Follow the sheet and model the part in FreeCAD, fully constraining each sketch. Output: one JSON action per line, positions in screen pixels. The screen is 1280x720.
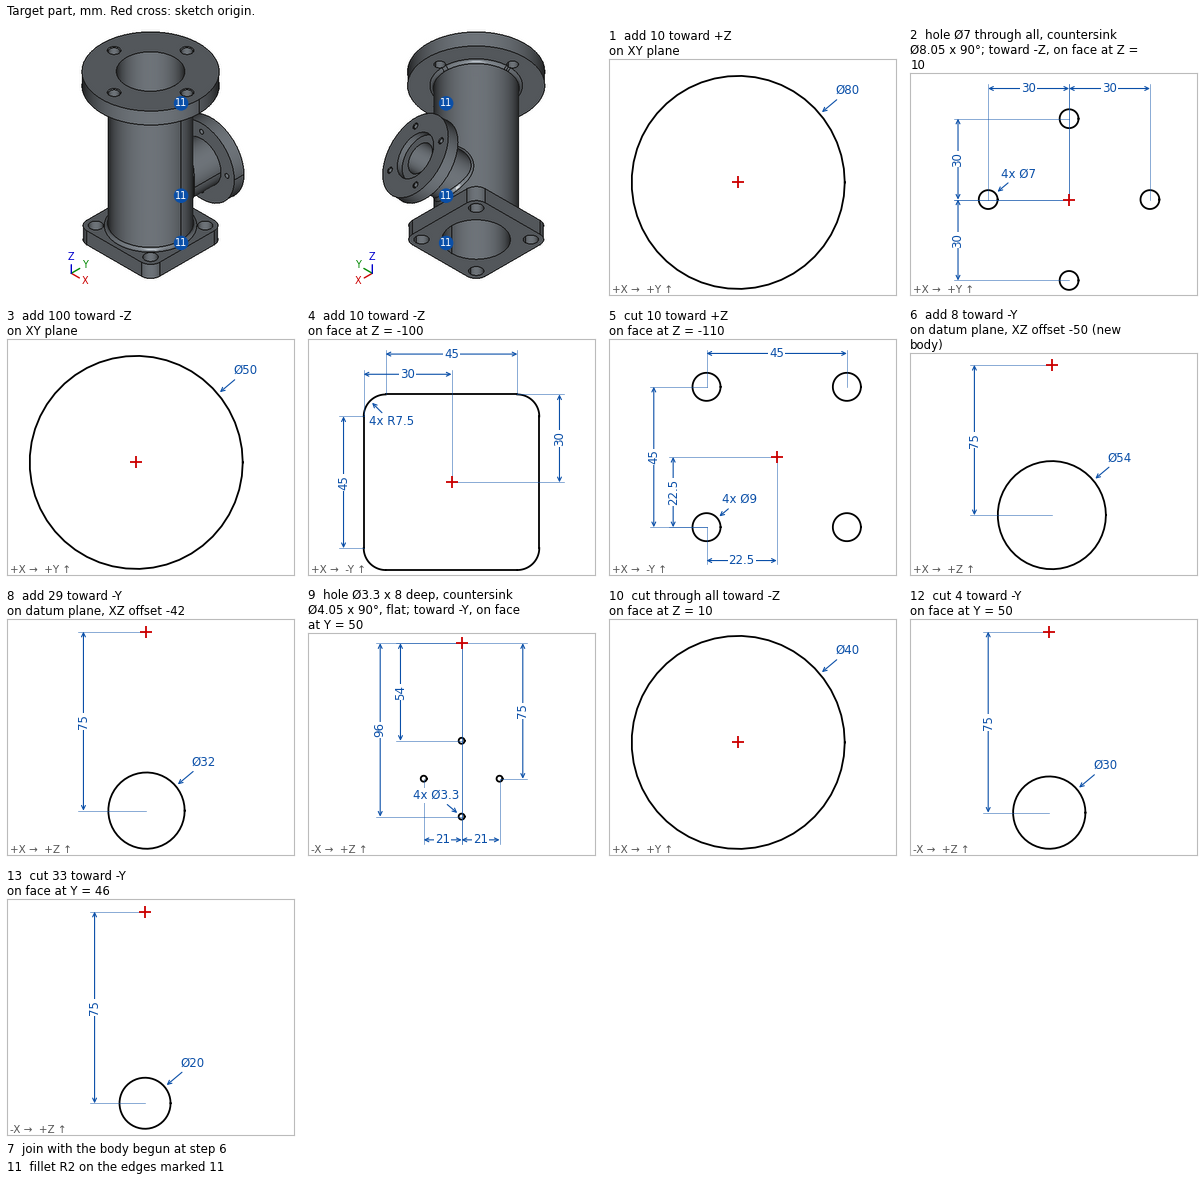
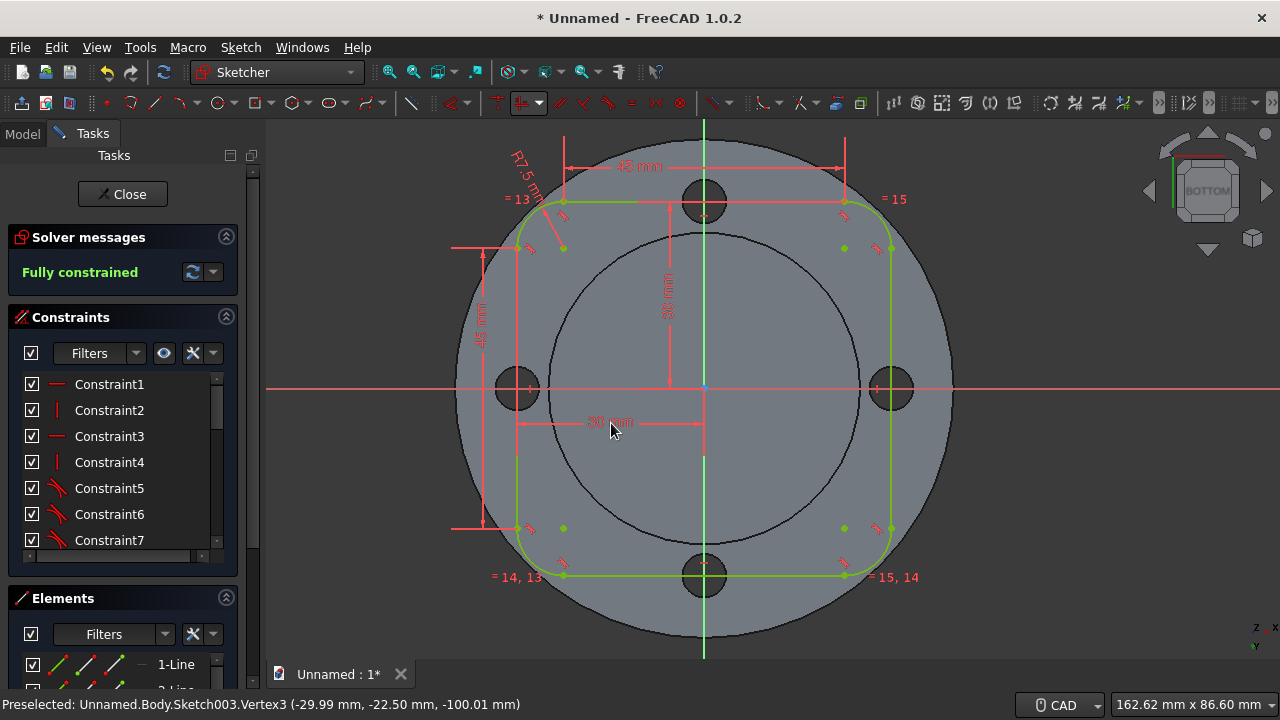
{"action": "left_click", "coordinate": [123, 194]}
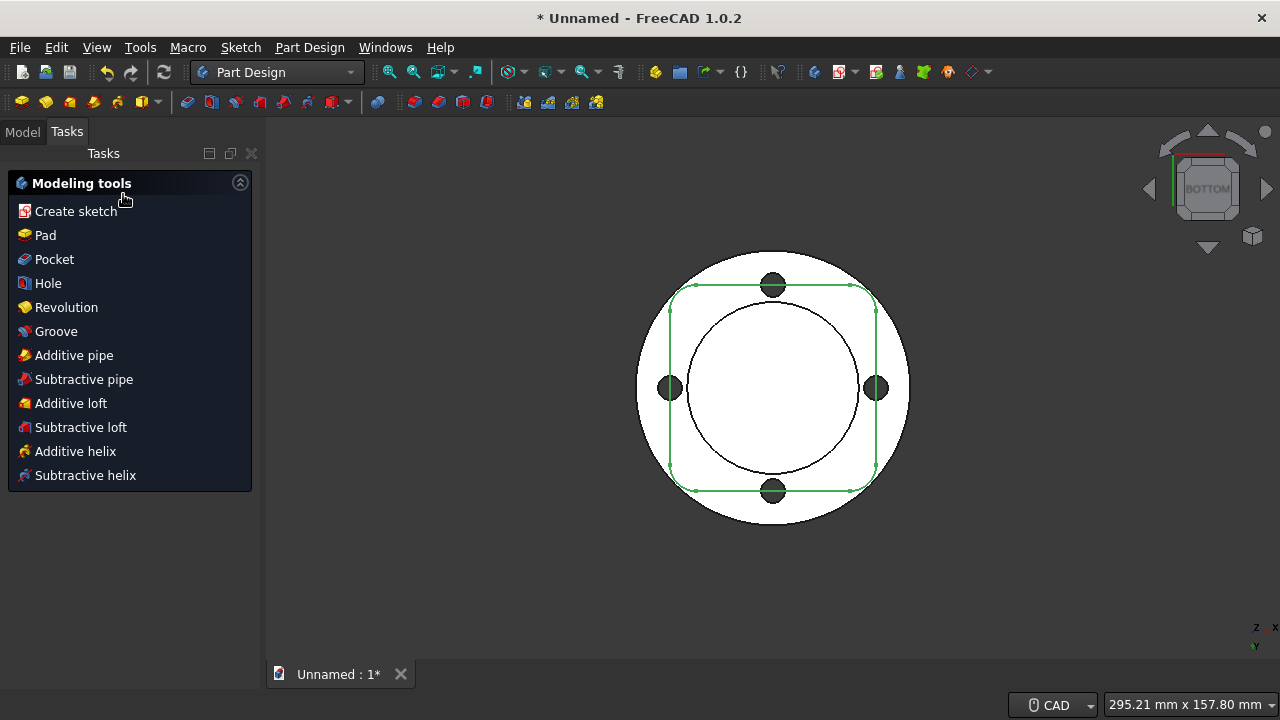
{"action": "left_click", "coordinate": [22, 102]}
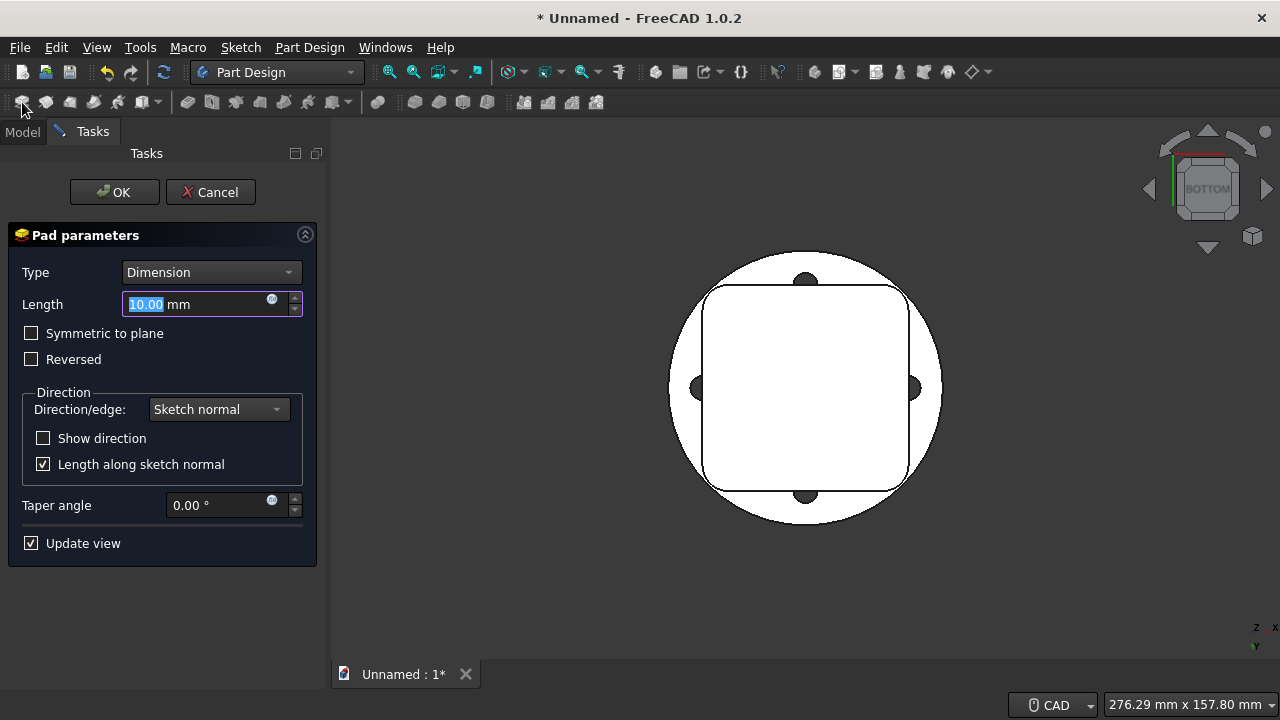
{"action": "type", "text": "10"}
{"action": "key", "text": "Tab"}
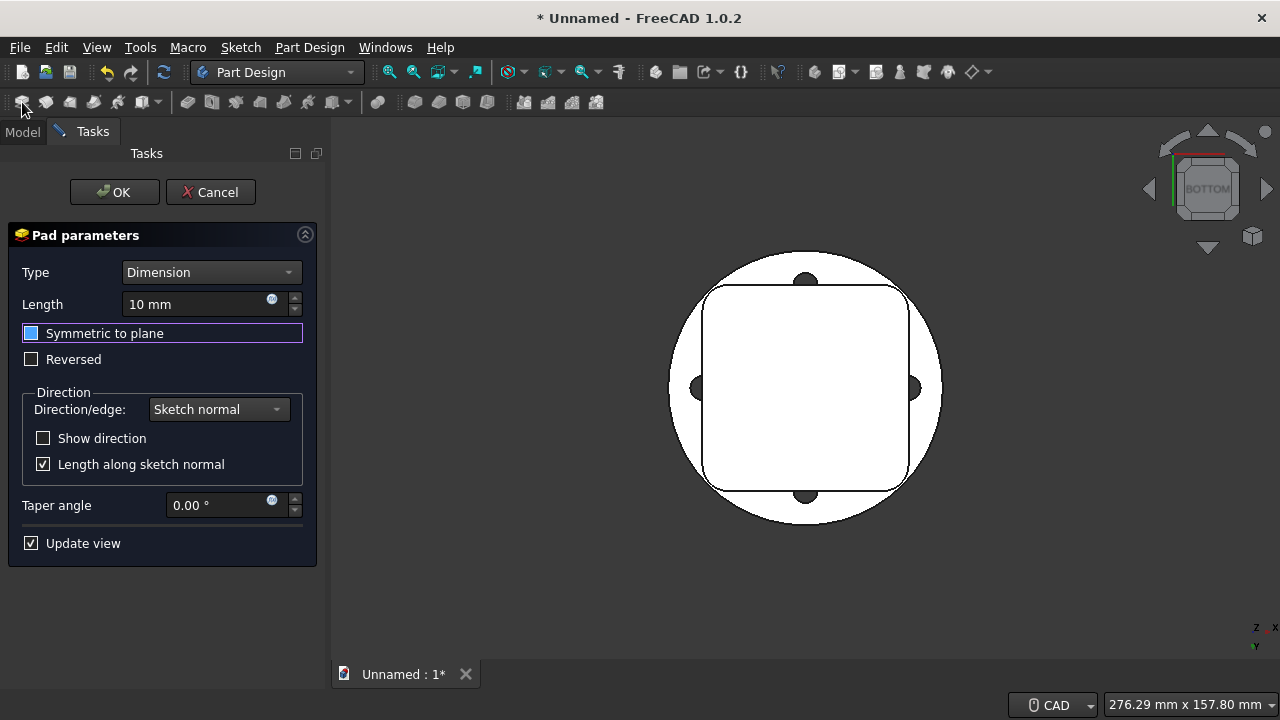
{"action": "left_click", "coordinate": [115, 192]}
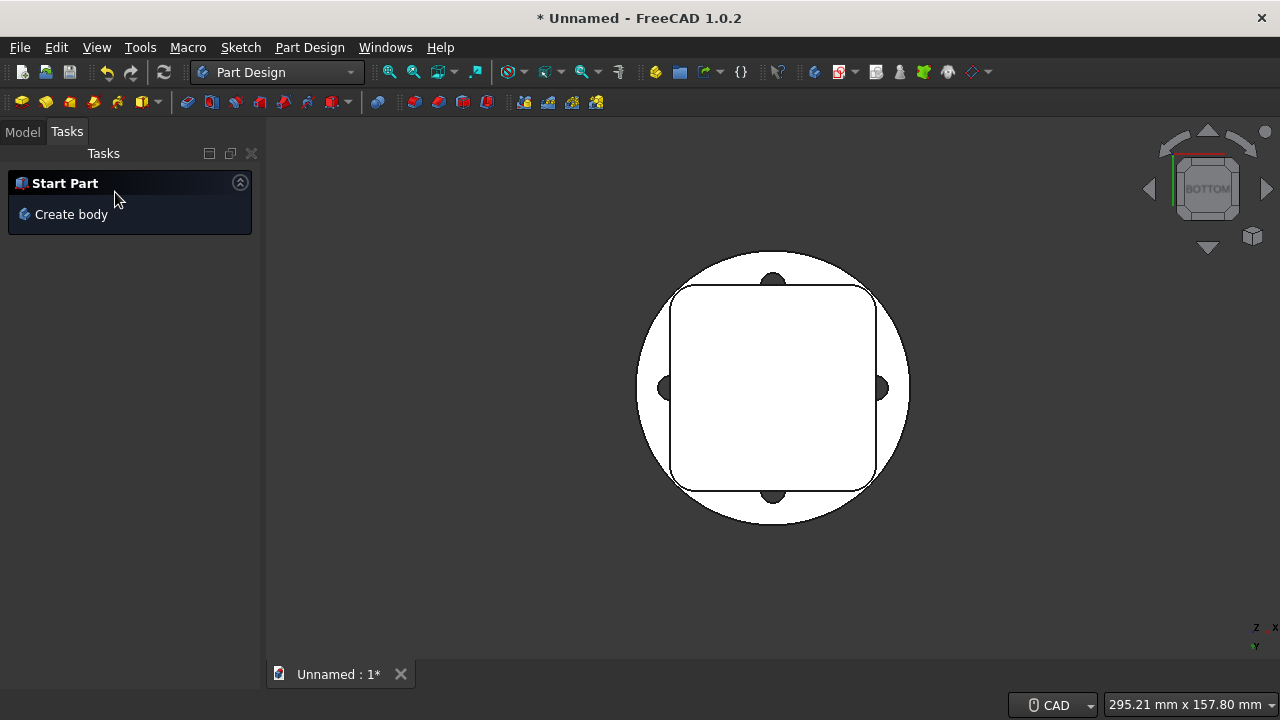
{"action": "left_click", "coordinate": [773, 387]}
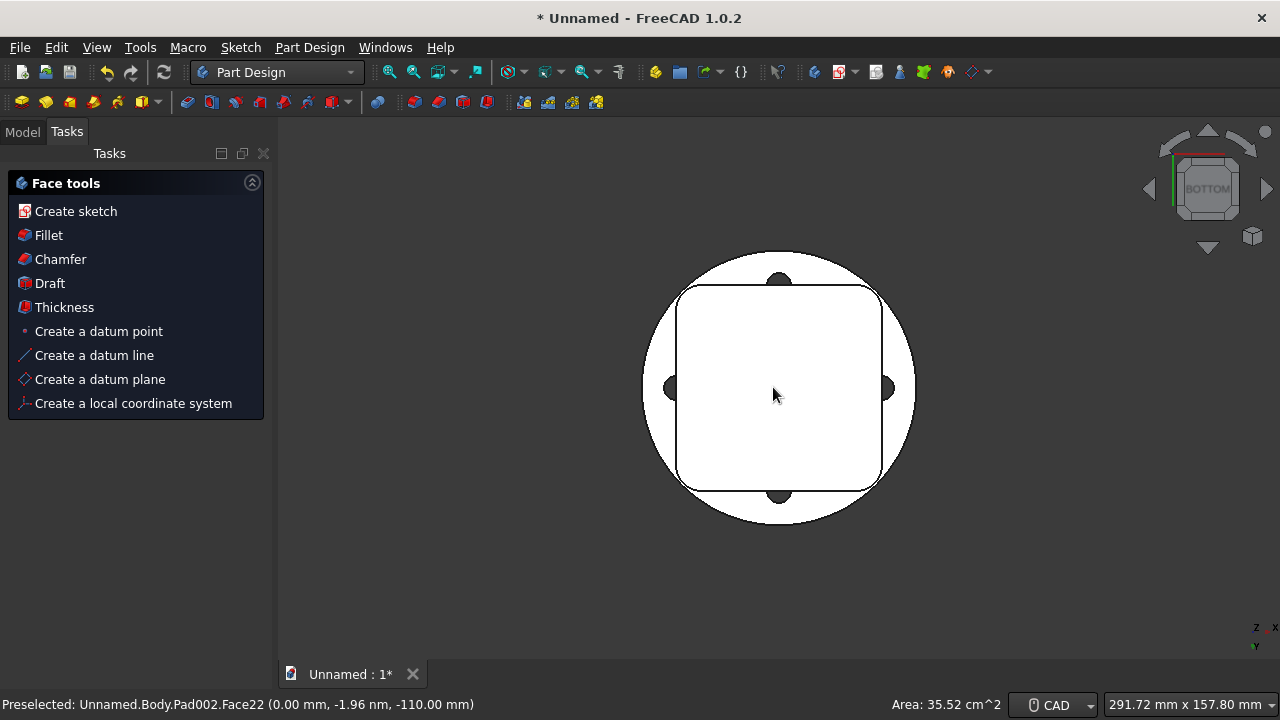
{"action": "left_click", "coordinate": [840, 72]}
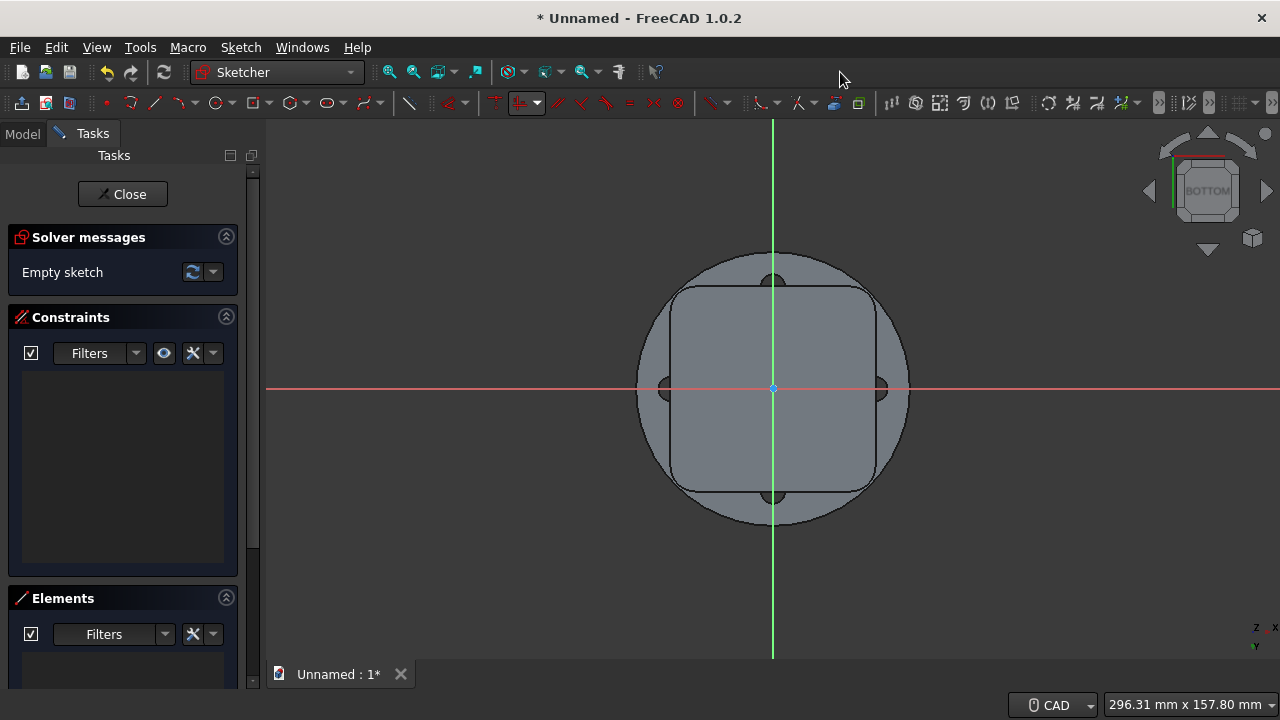
{"action": "scroll", "coordinate": [856, 389], "scroll_direction": "up", "scroll_amount": 3}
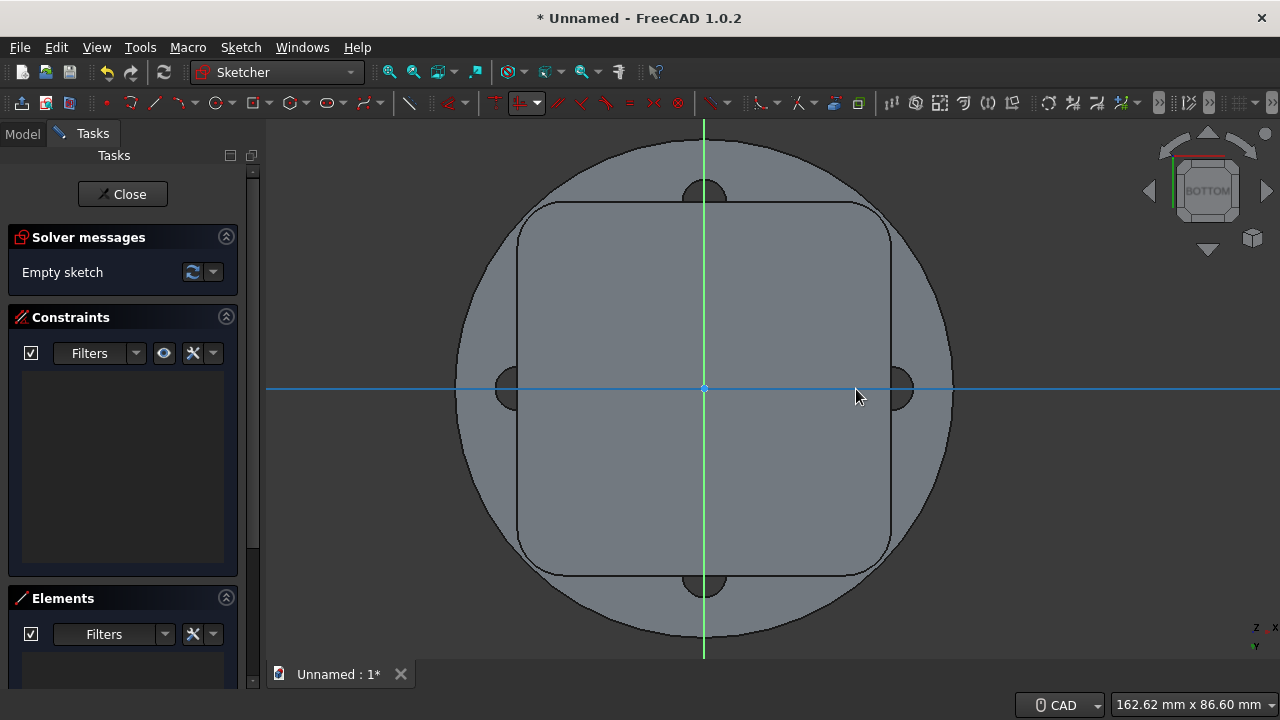
{"action": "left_click", "coordinate": [216, 104]}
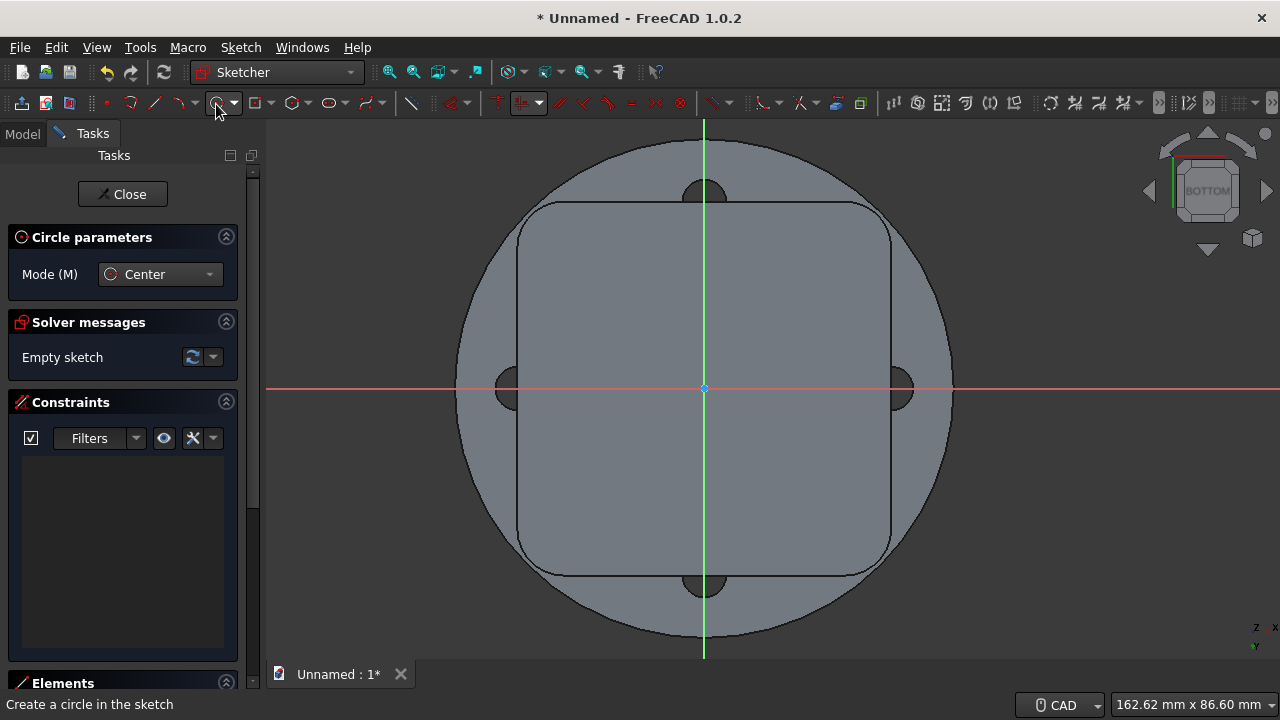
{"action": "left_click", "coordinate": [564, 529]}
{"action": "mouse_move", "coordinate": [584, 509]}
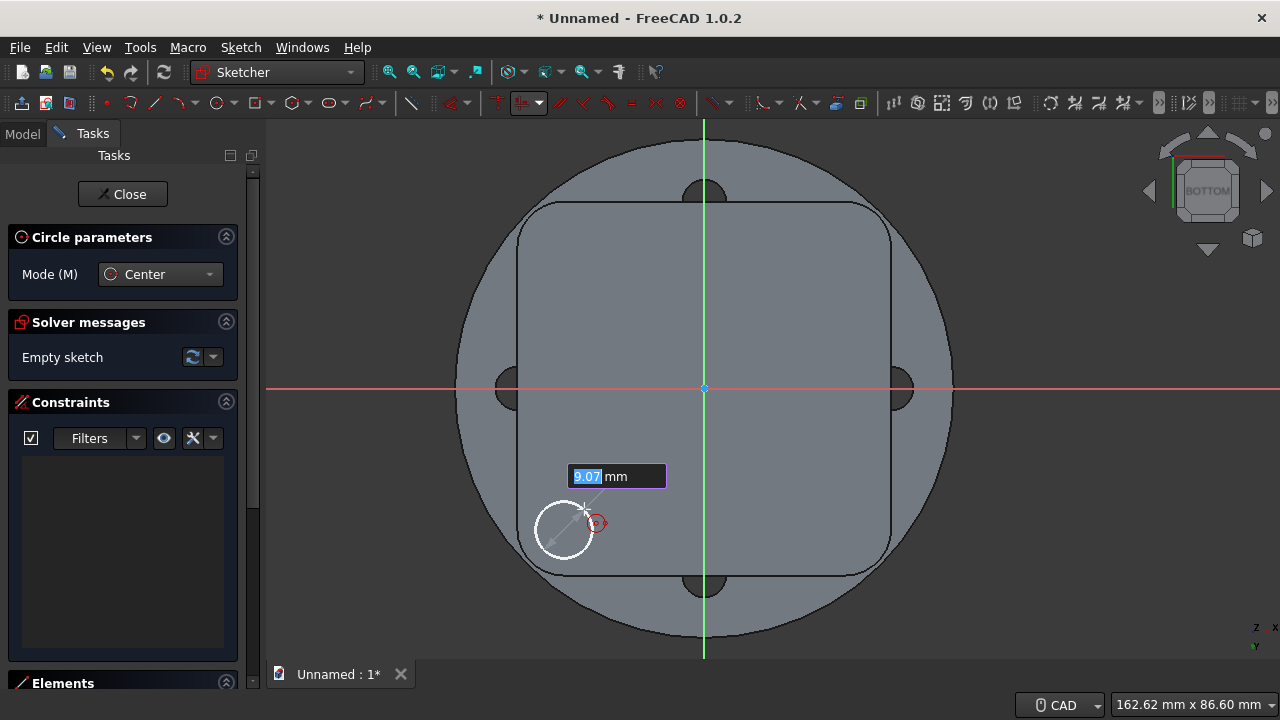
{"action": "type", "text": "9"}
{"action": "key", "text": "Return"}